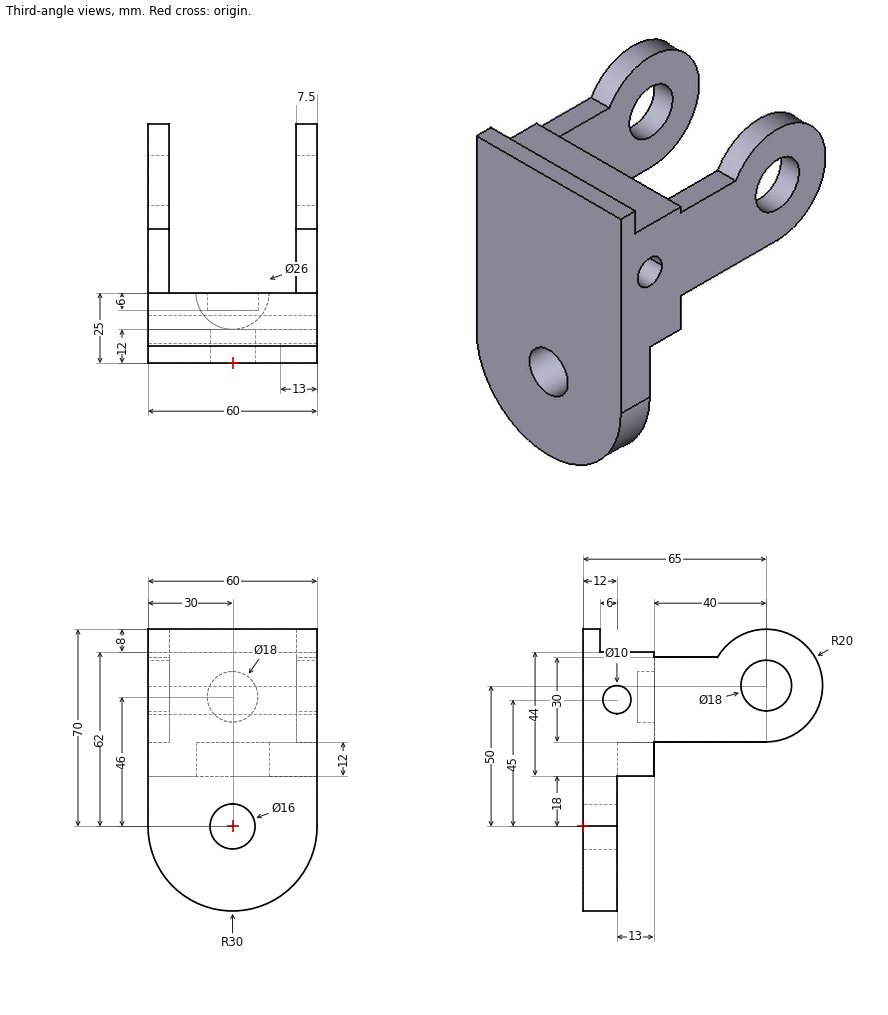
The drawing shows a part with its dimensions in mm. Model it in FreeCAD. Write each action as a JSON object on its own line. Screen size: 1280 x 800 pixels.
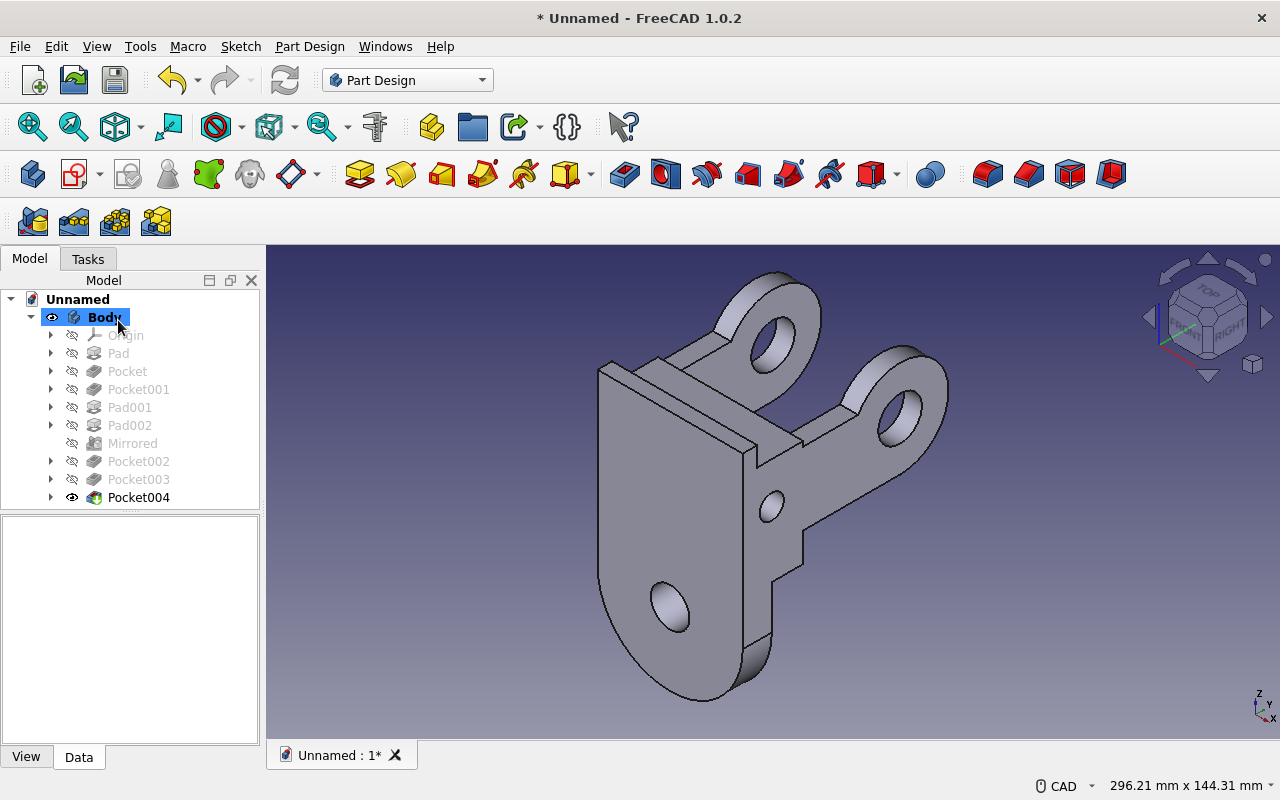
{"action": "left_click", "coordinate": [51, 335]}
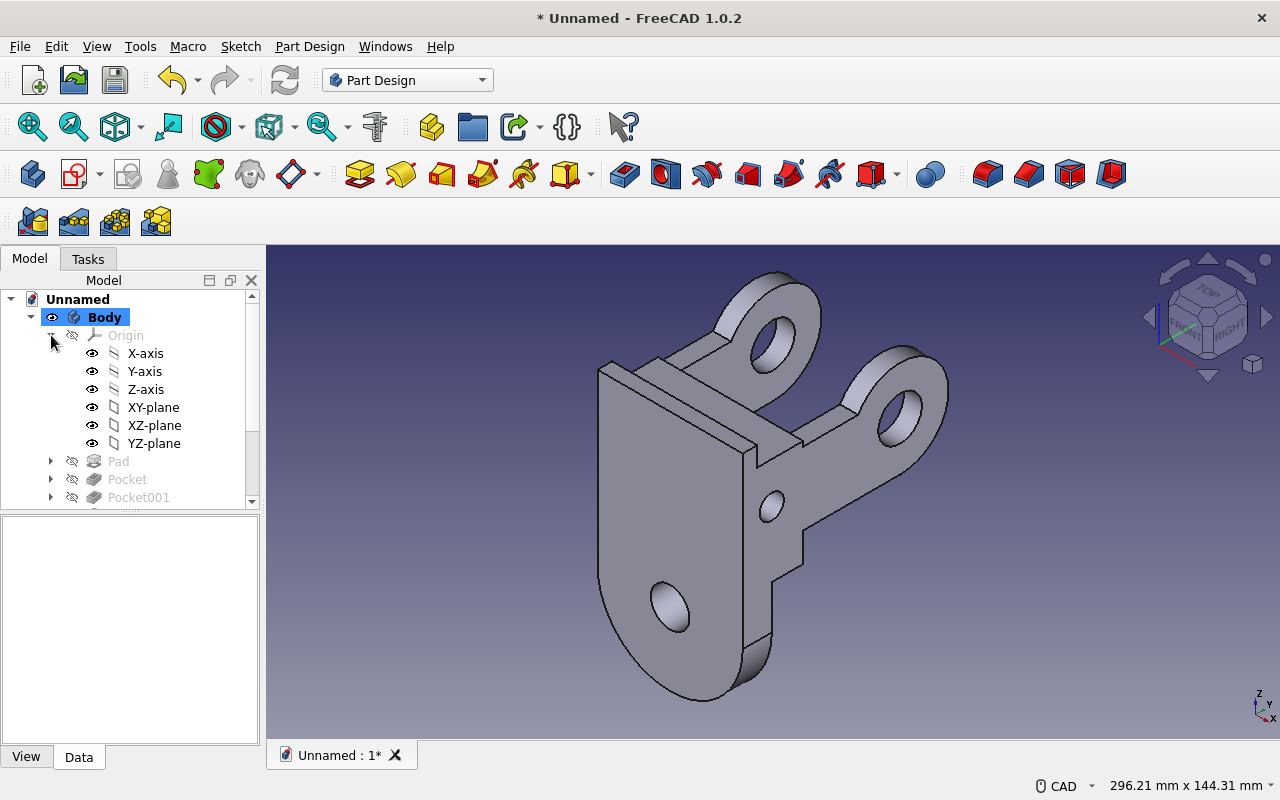
{"action": "left_click", "coordinate": [137, 443]}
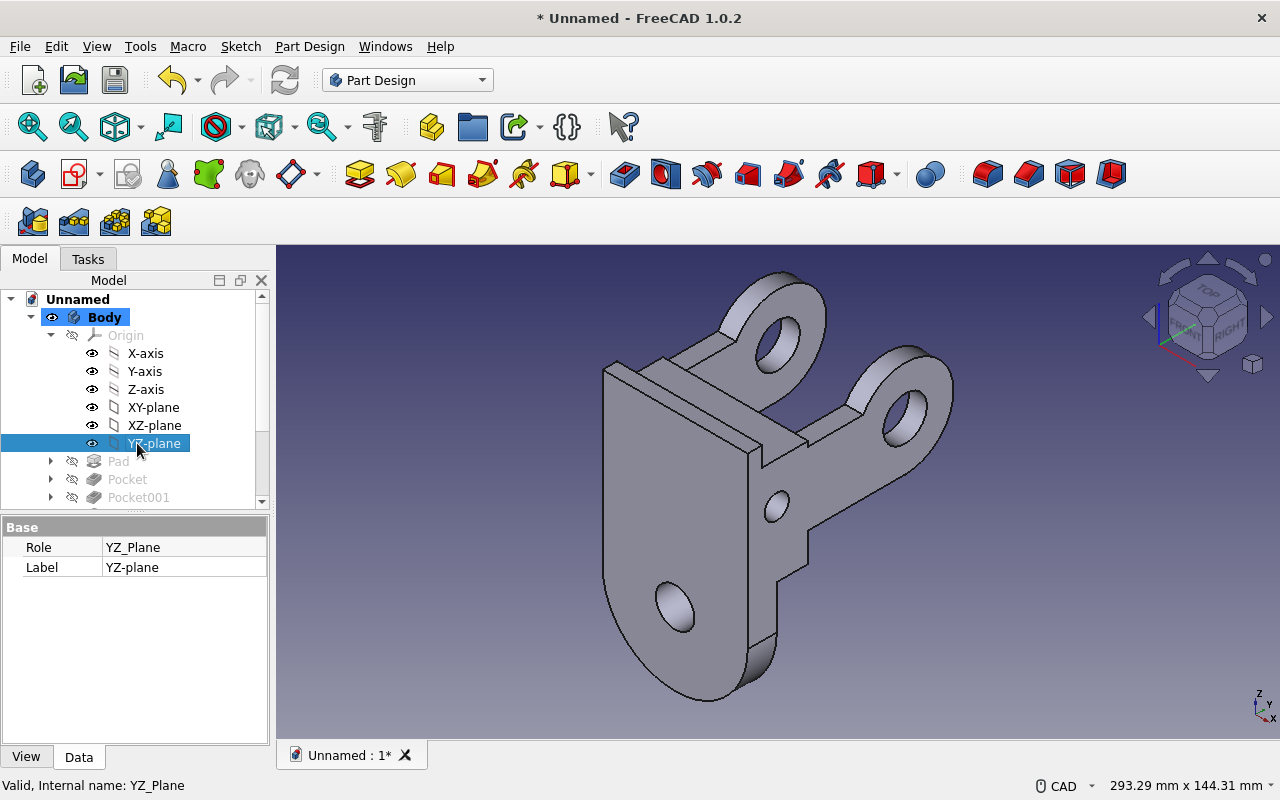
{"action": "left_click", "coordinate": [290, 174]}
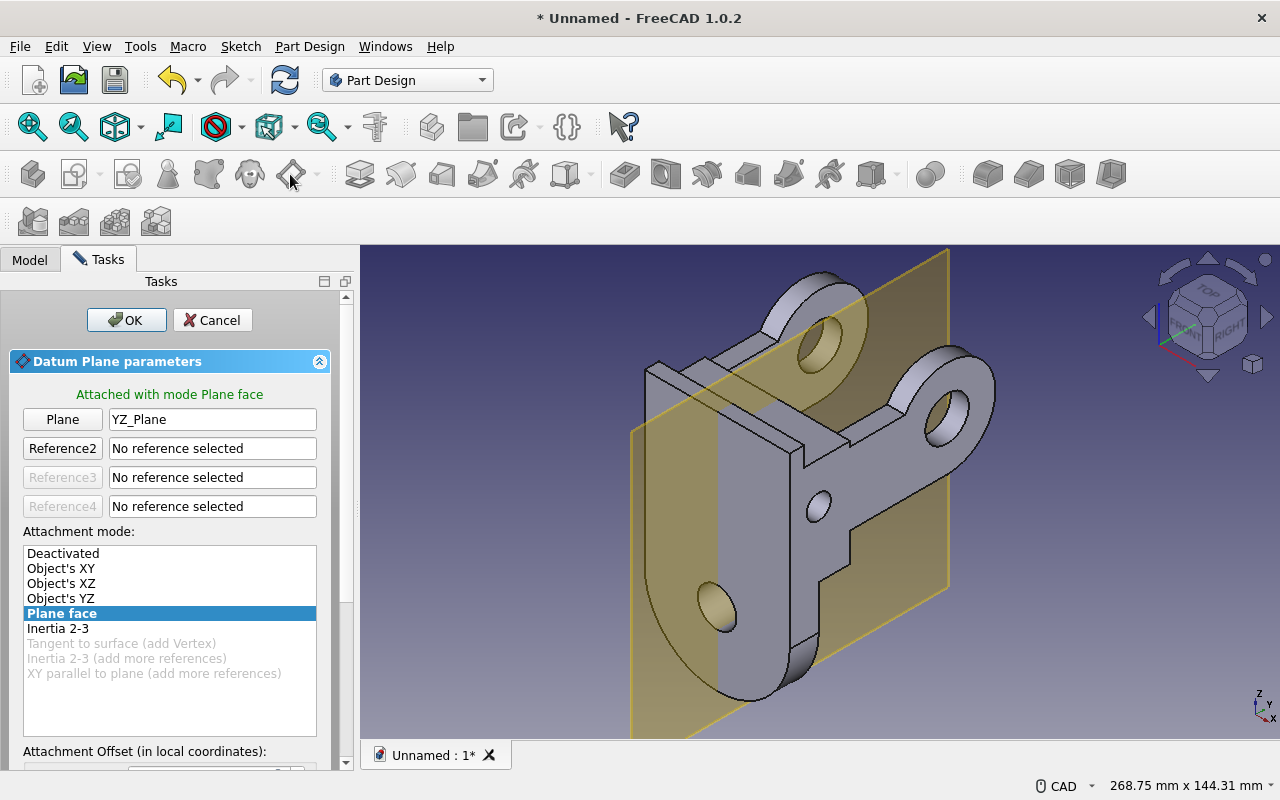
{"action": "scroll", "coordinate": [346, 530], "scroll_direction": "down", "scroll_amount": 3}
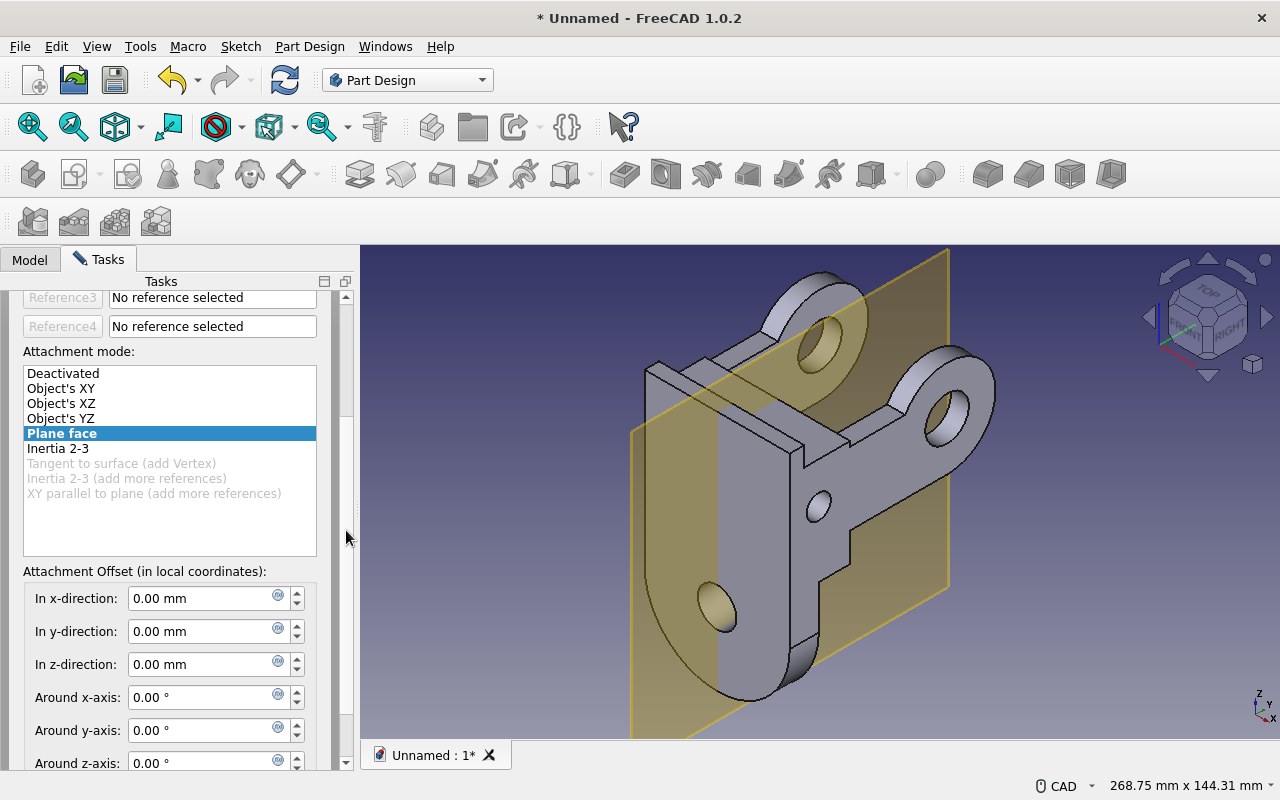
{"action": "triple_click", "coordinate": [210, 664]}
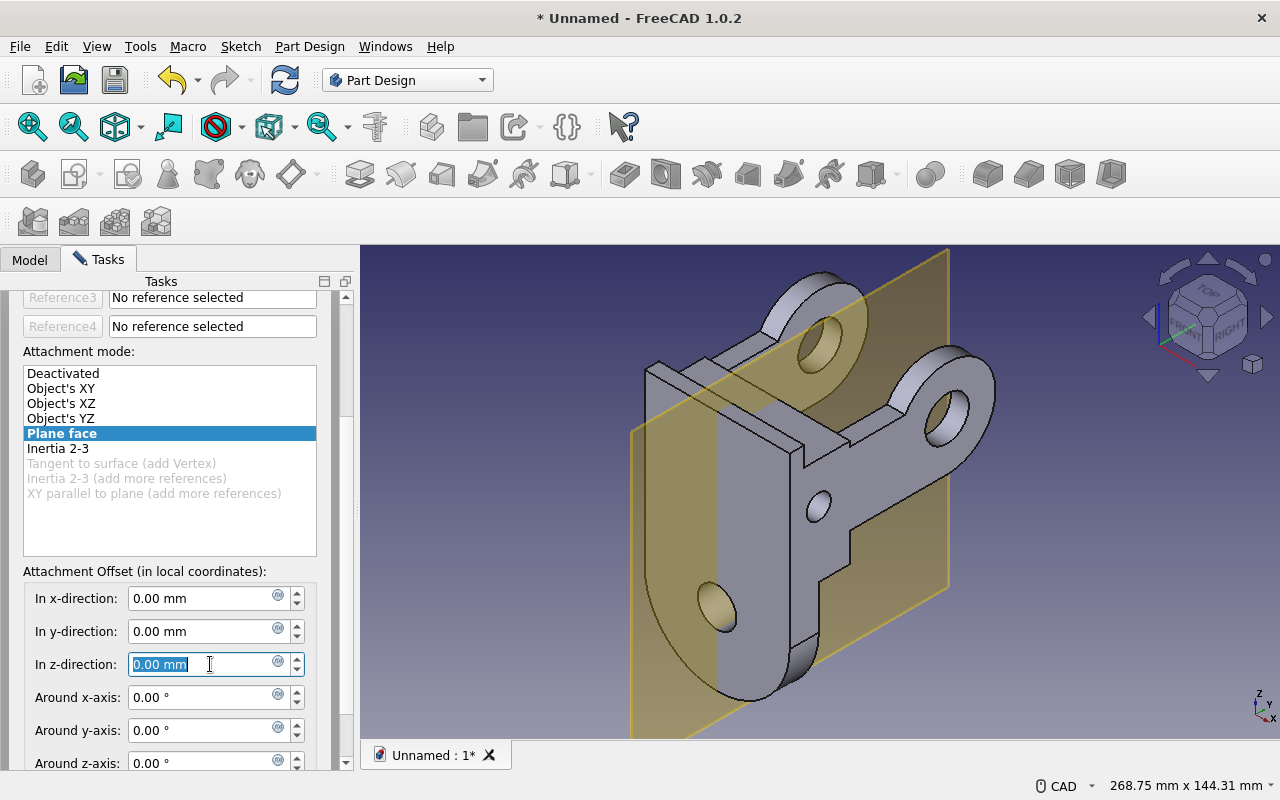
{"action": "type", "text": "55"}
{"action": "key", "text": "Tab"}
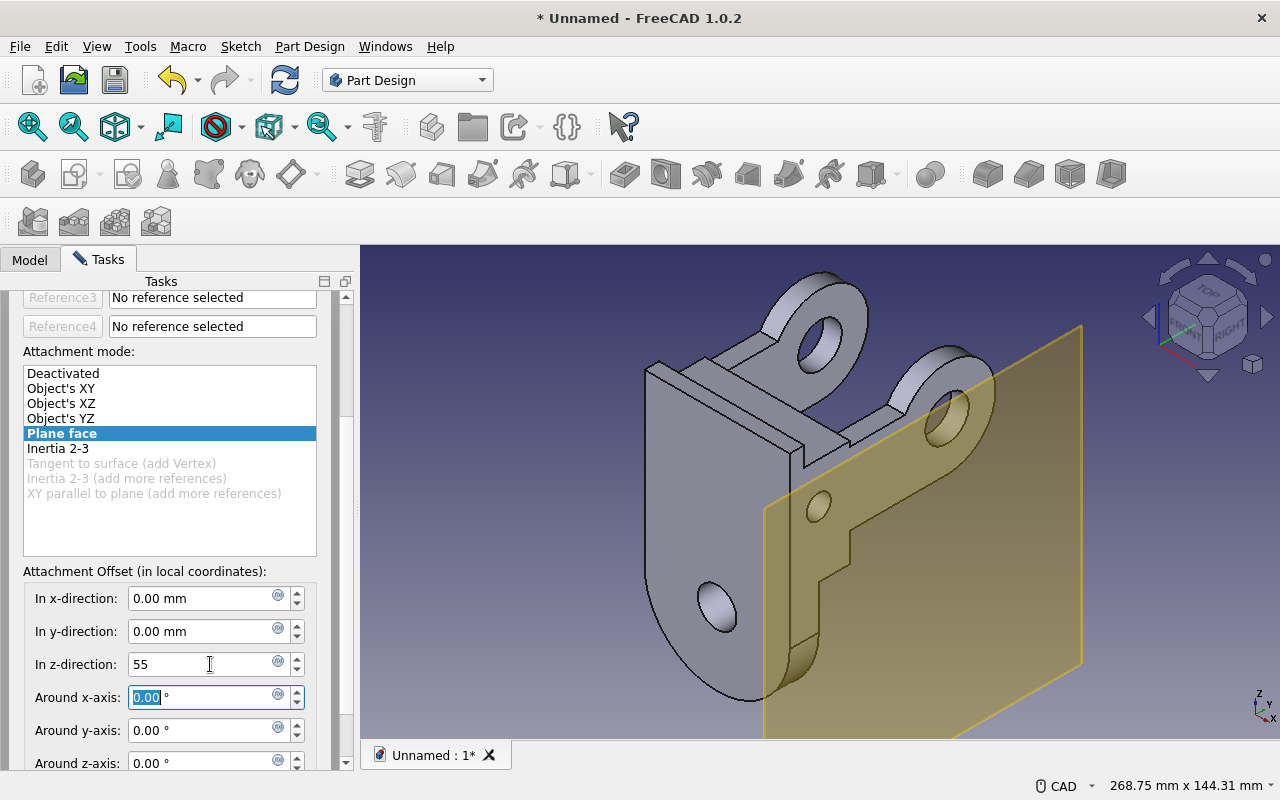
{"action": "scroll", "coordinate": [346, 530], "scroll_direction": "up", "scroll_amount": 4}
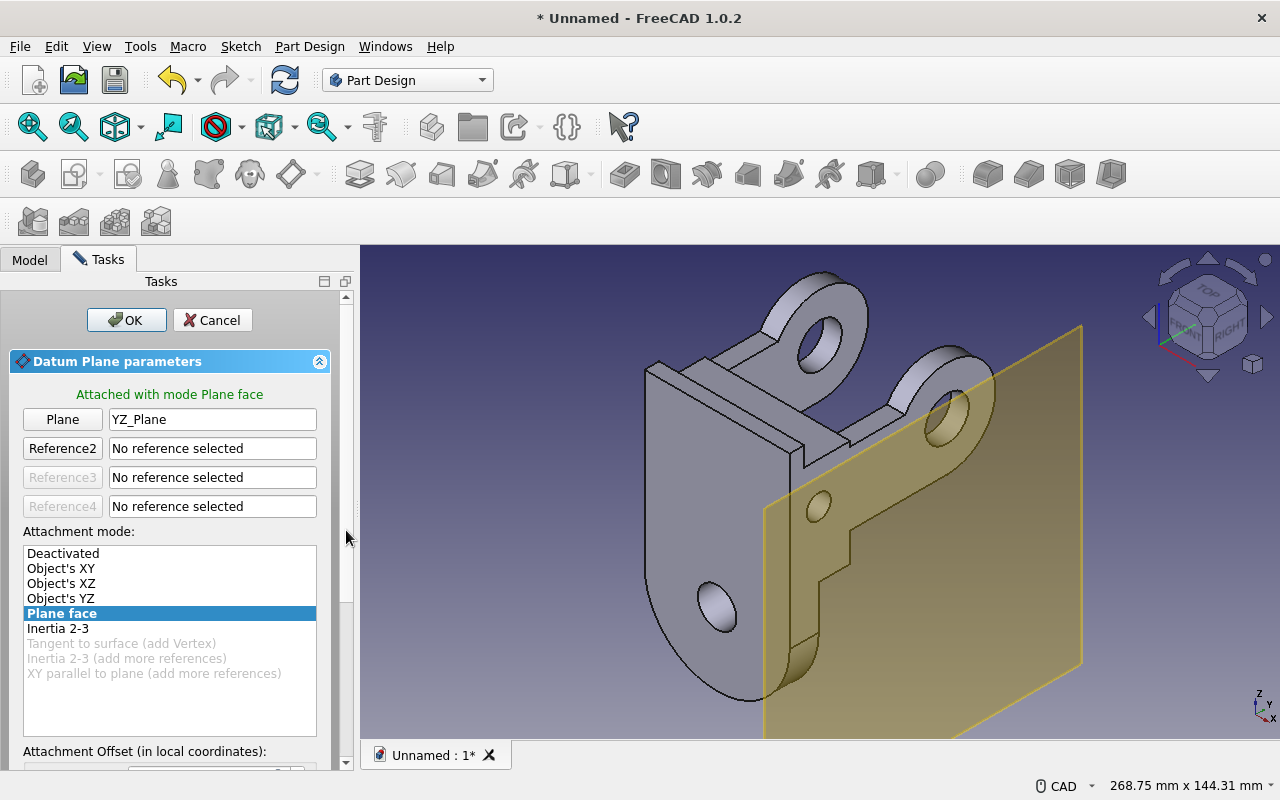
{"action": "left_click", "coordinate": [127, 320]}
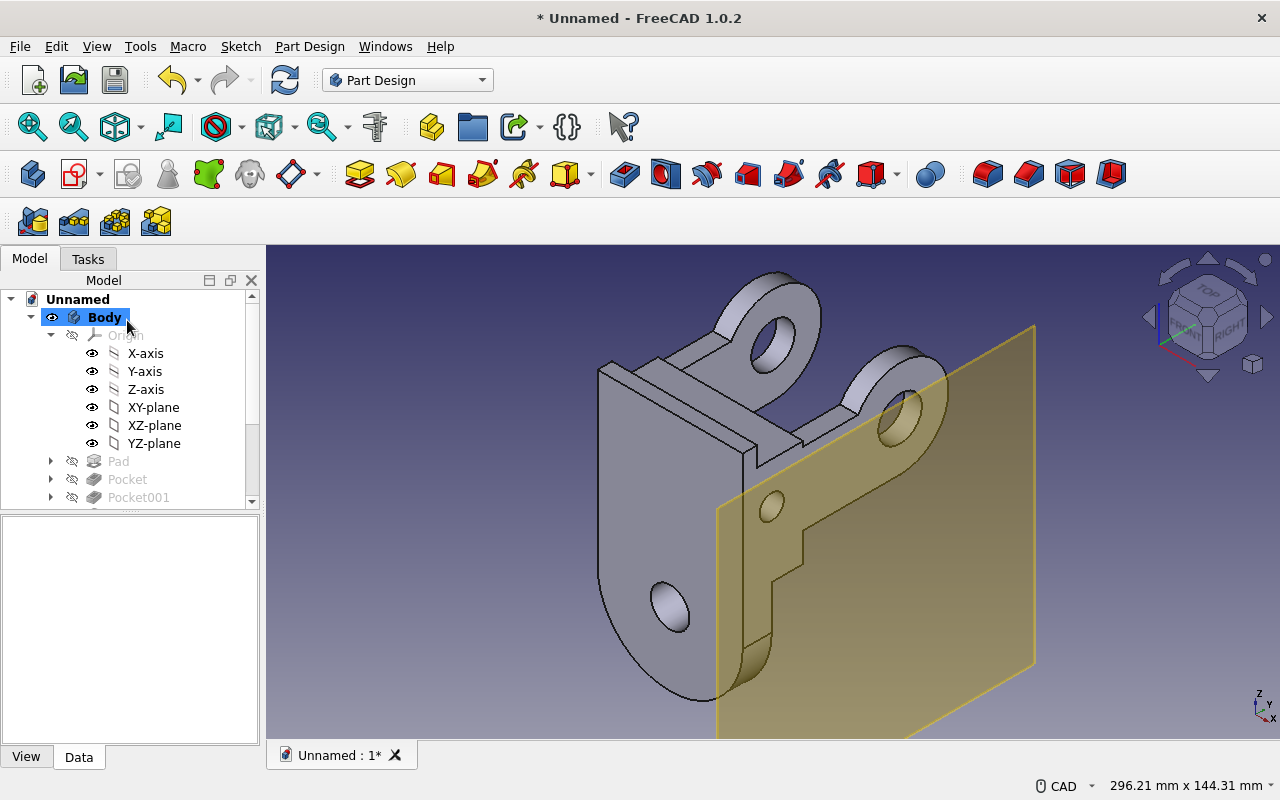
{"action": "scroll", "coordinate": [101, 403], "scroll_direction": "down", "scroll_amount": 3}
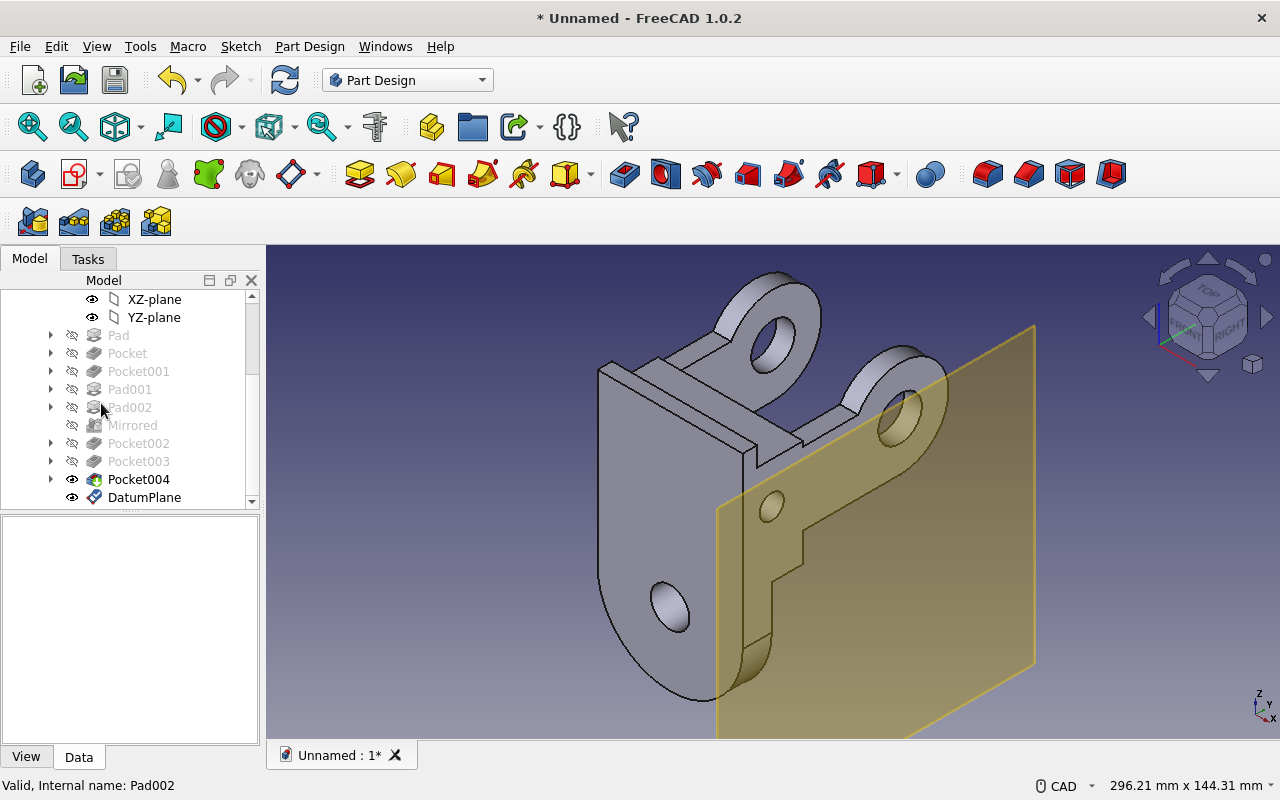
{"action": "left_click", "coordinate": [117, 497]}